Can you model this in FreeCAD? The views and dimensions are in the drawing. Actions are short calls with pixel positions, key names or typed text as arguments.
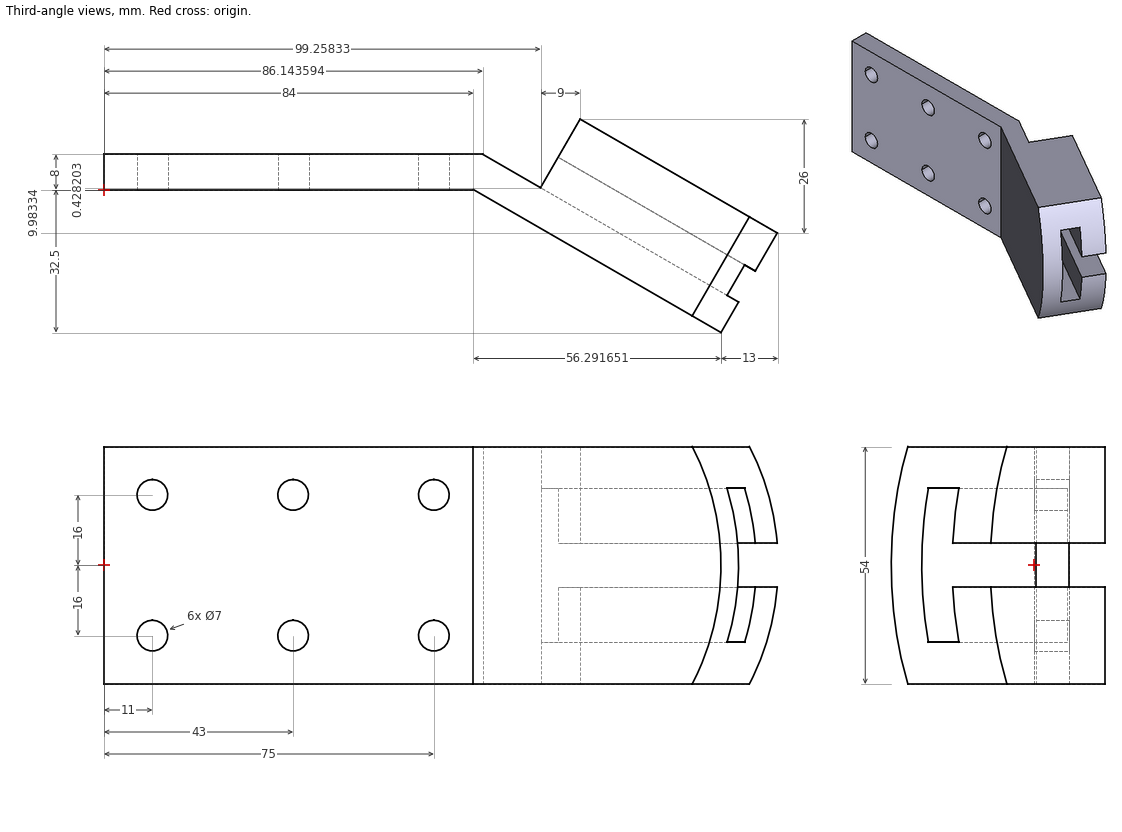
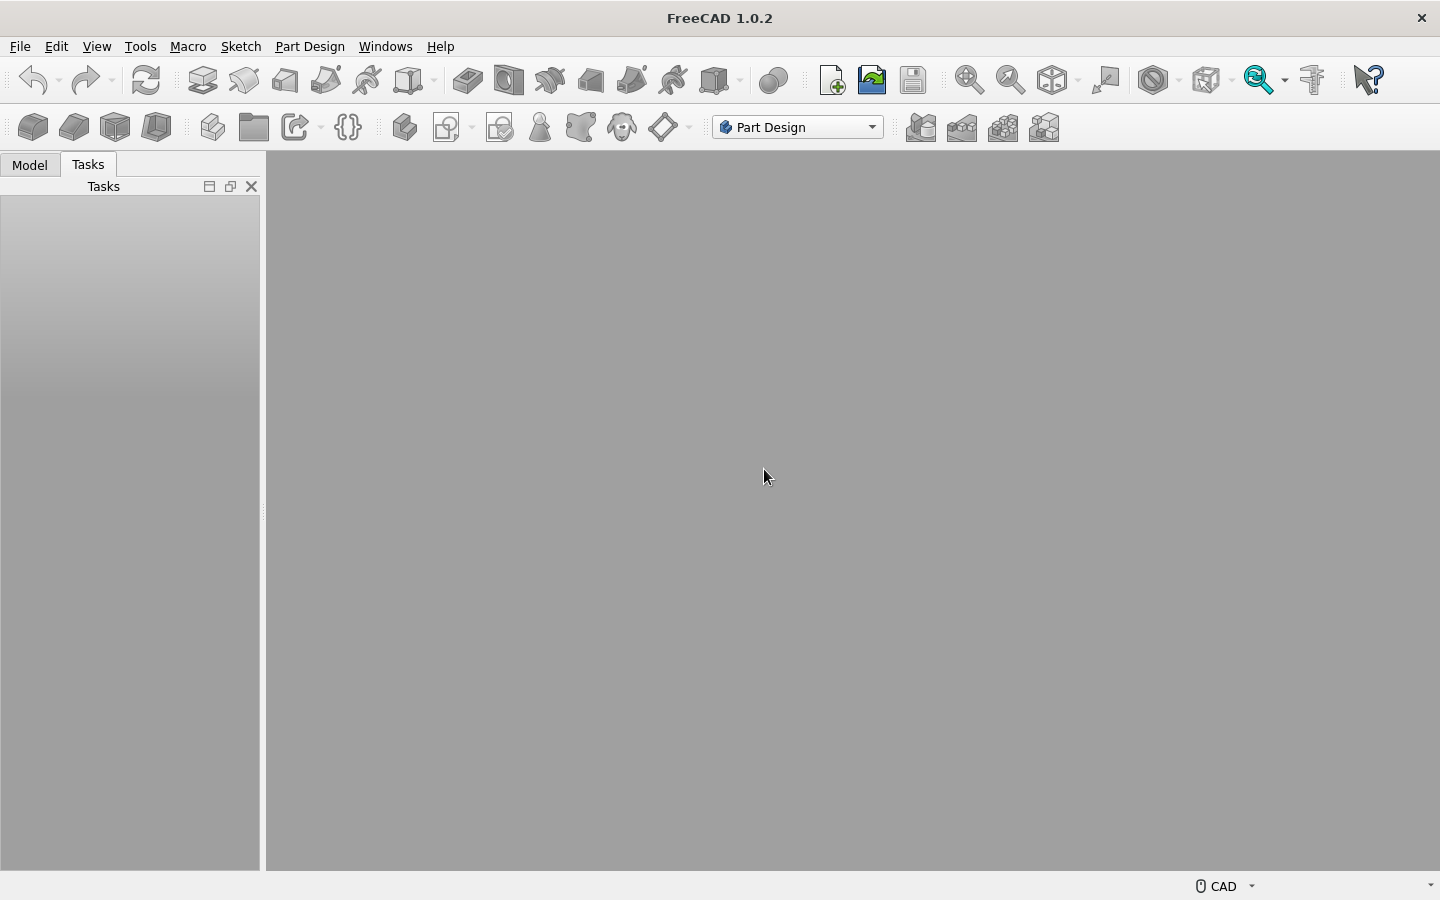
key(ctrl+n)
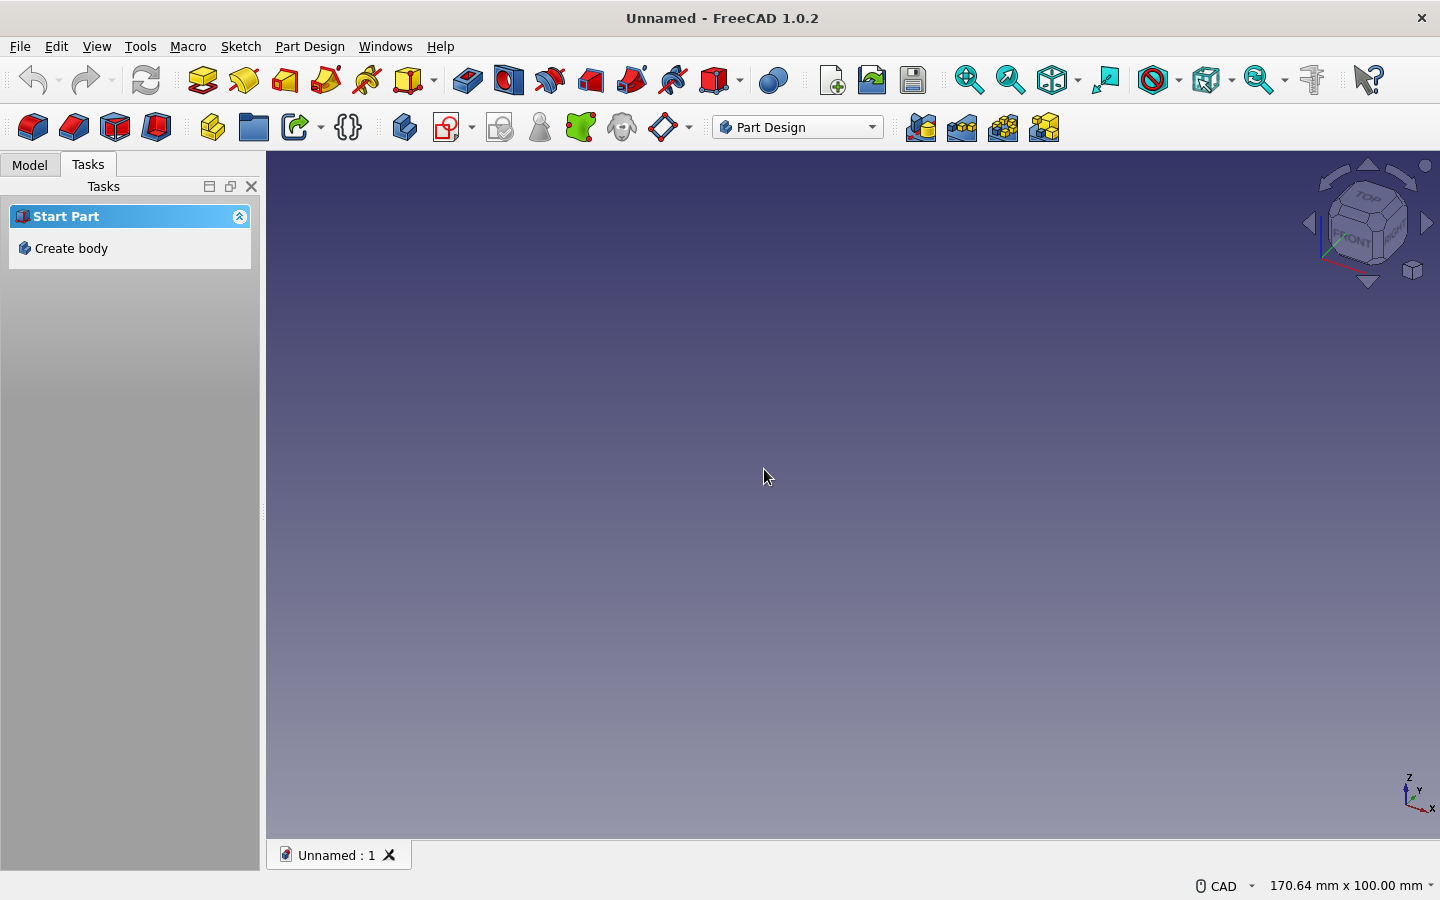
click(446, 128)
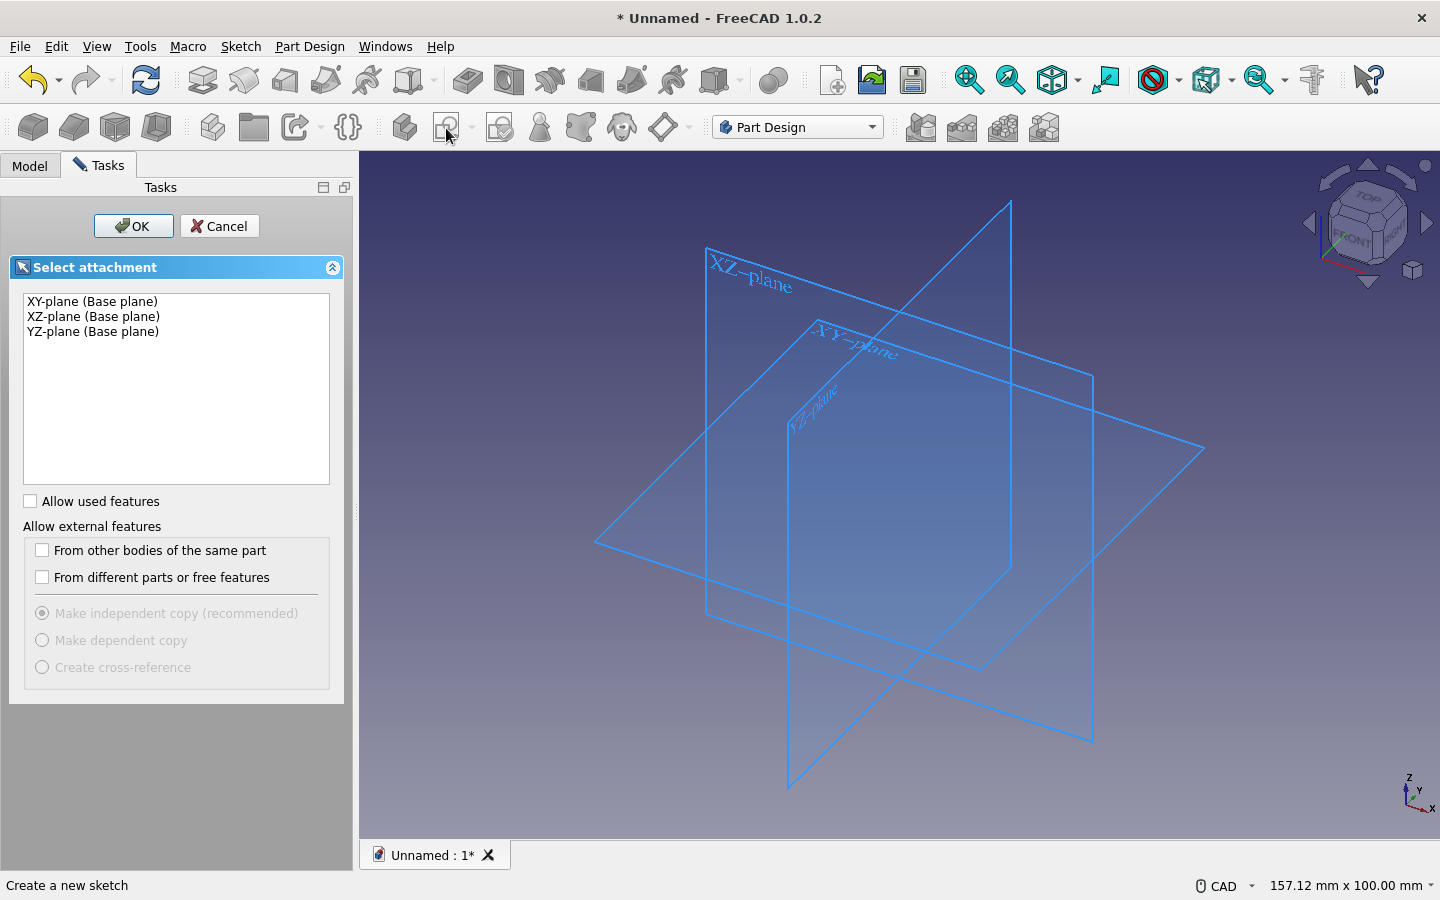
click(84, 302)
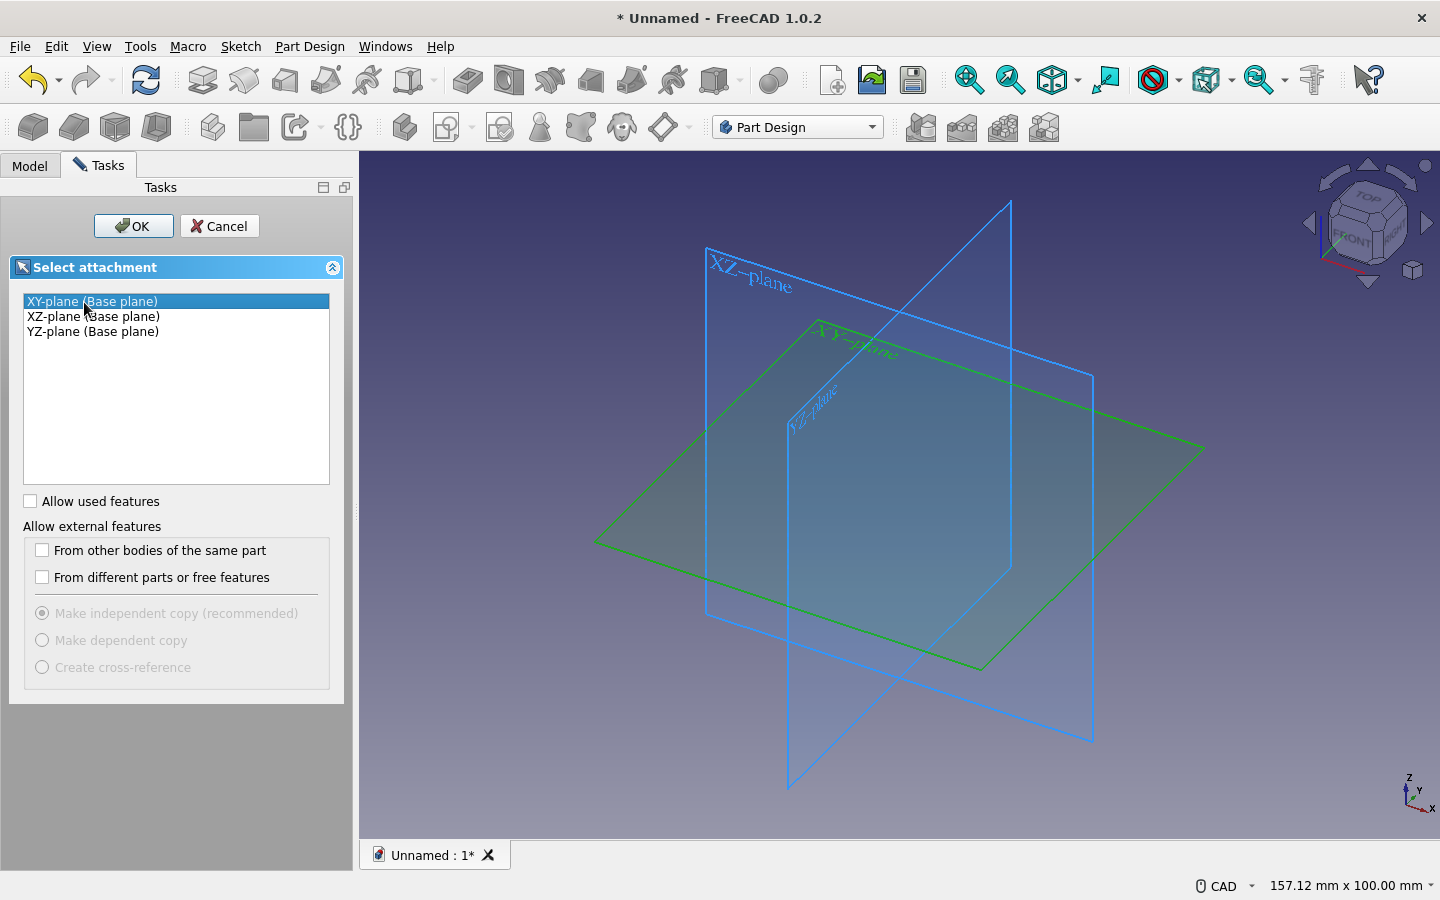
click(134, 226)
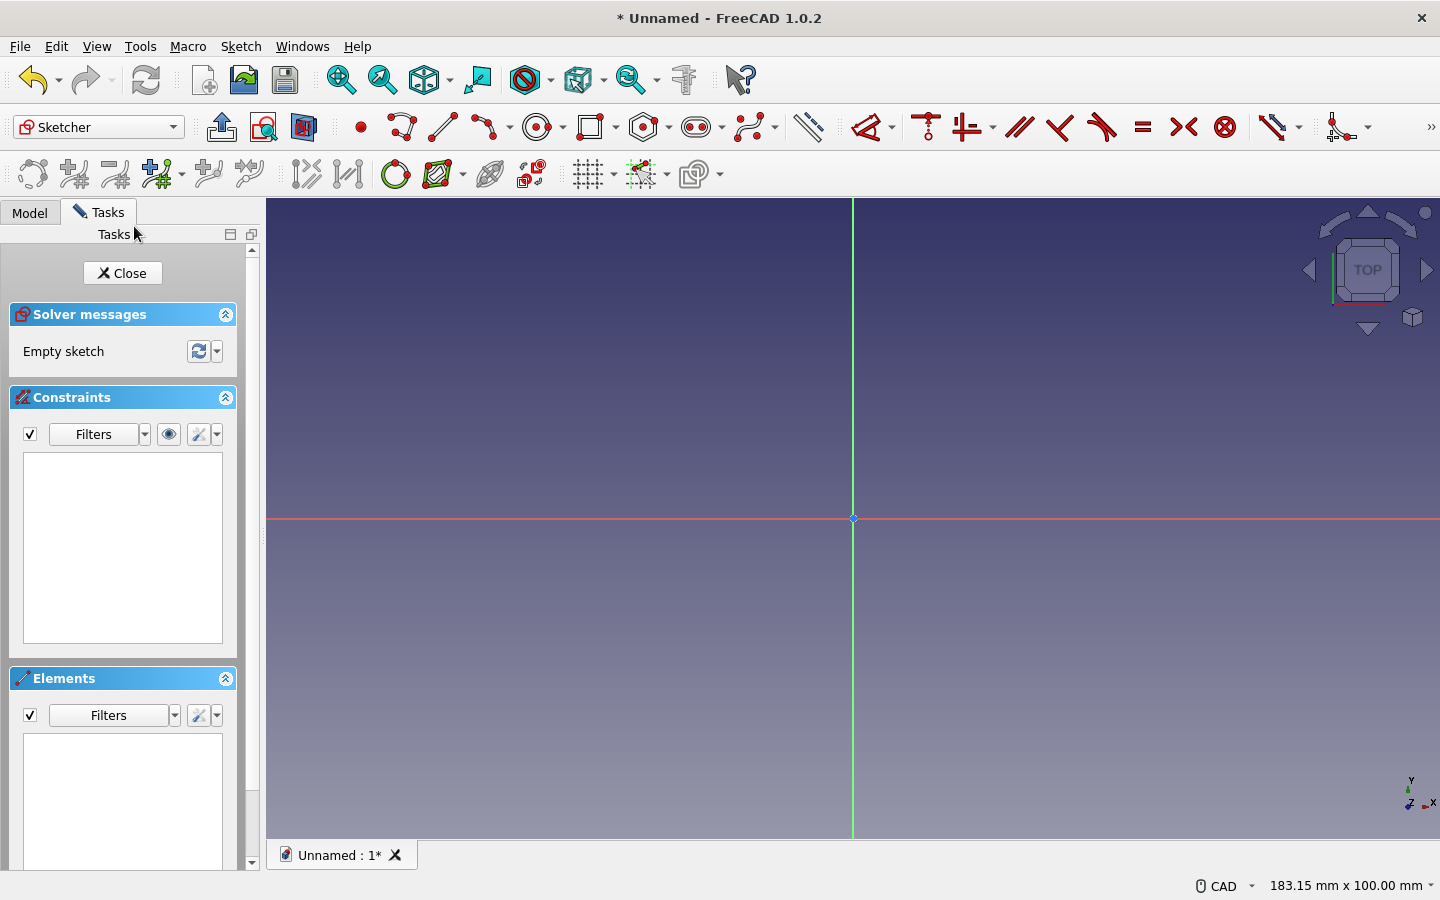
scroll(294, 454, down, 3)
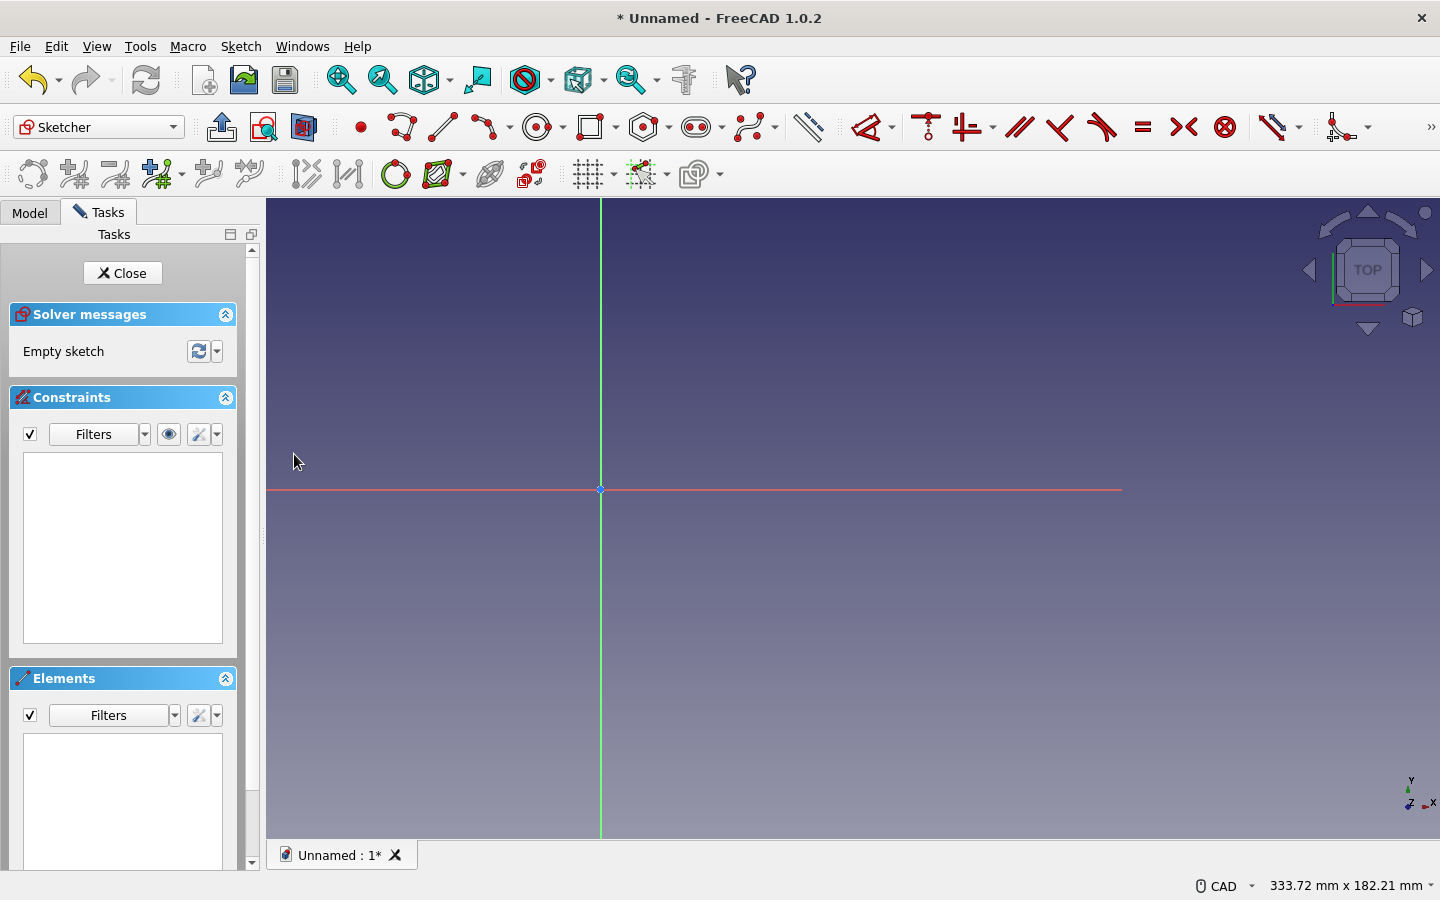
key(g)
key(m)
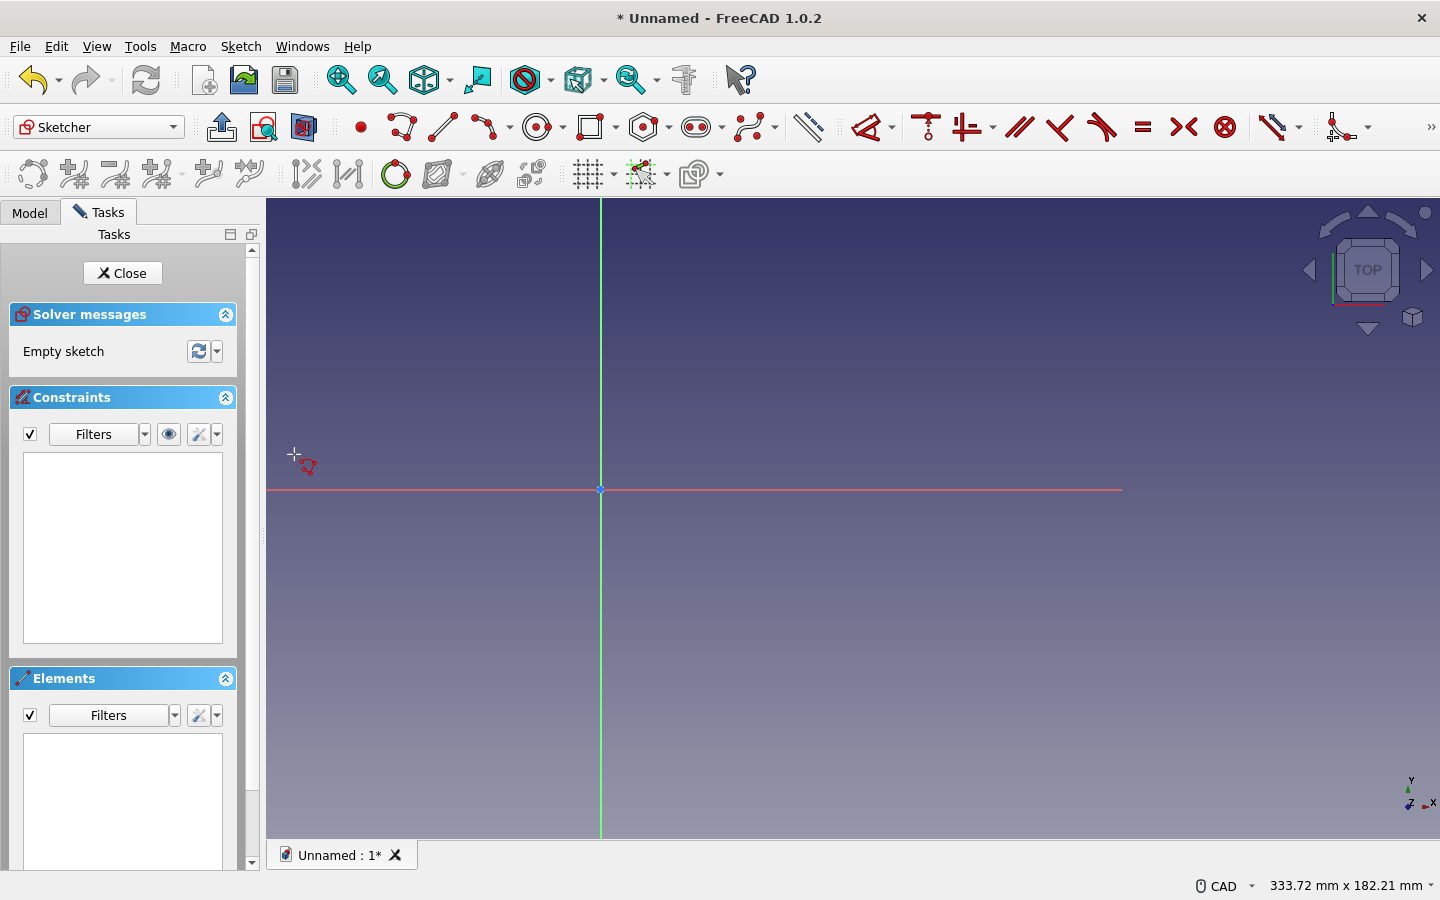
click(601, 490)
click(896, 499)
click(1094, 604)
click(1140, 525)
click(982, 433)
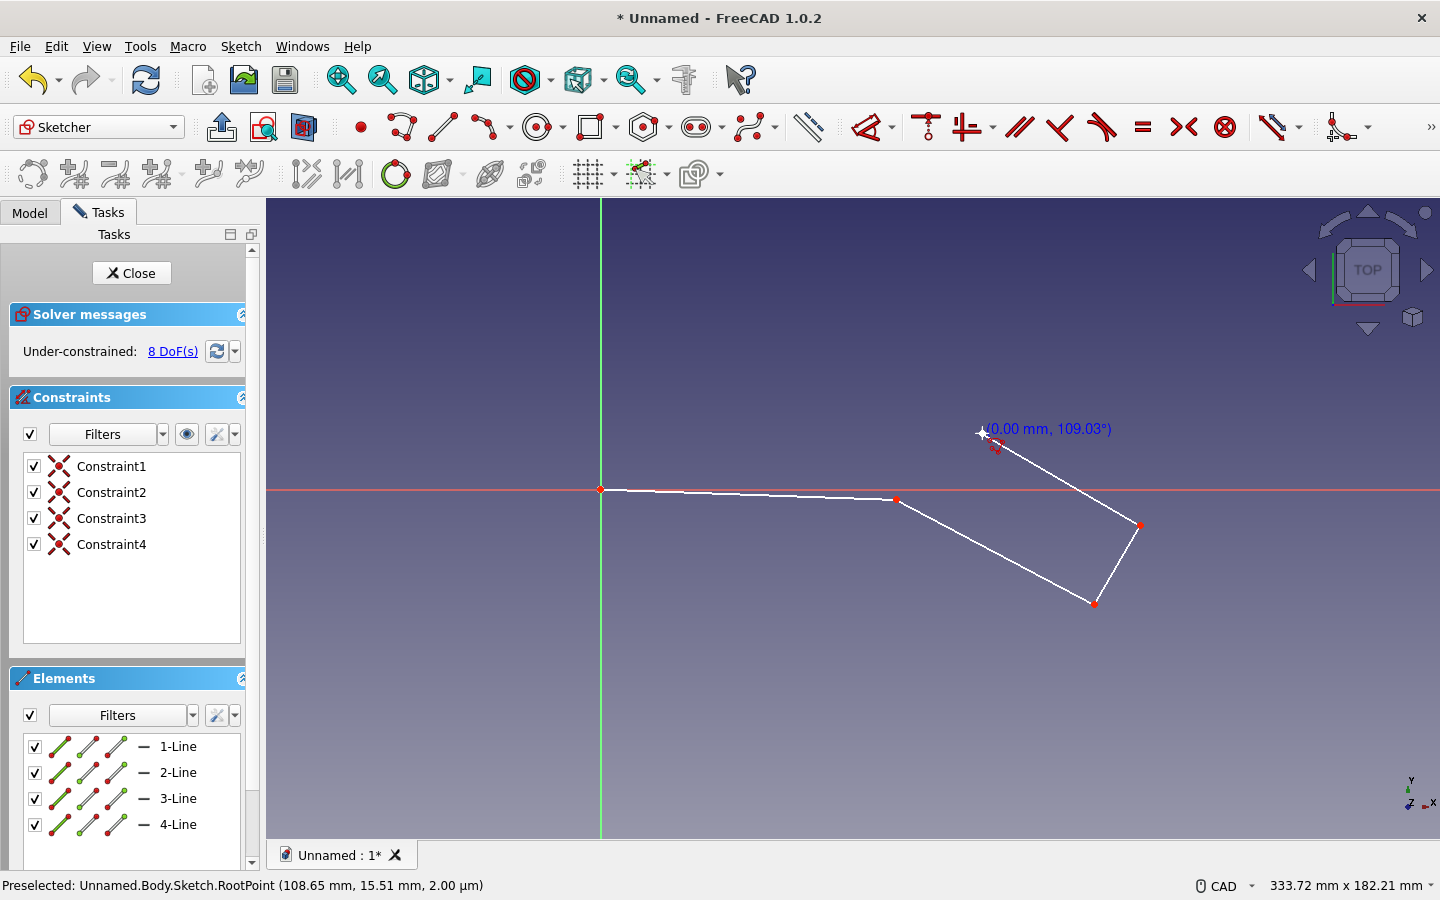
scroll(950, 488, up, 12)